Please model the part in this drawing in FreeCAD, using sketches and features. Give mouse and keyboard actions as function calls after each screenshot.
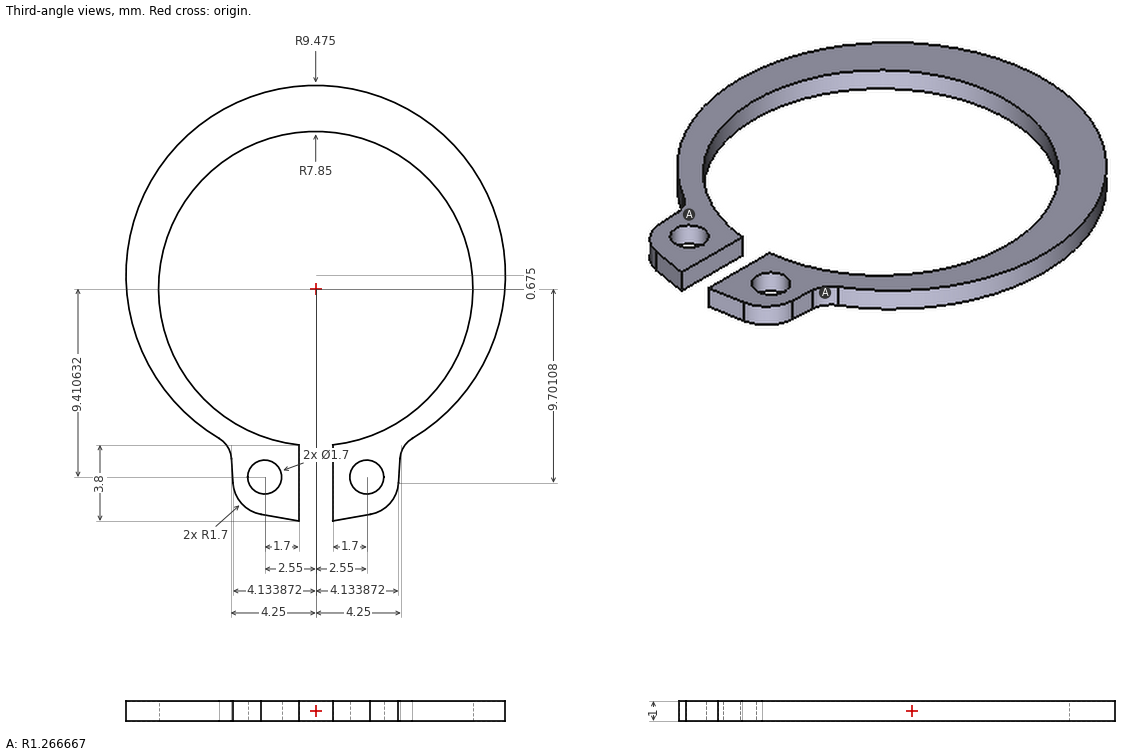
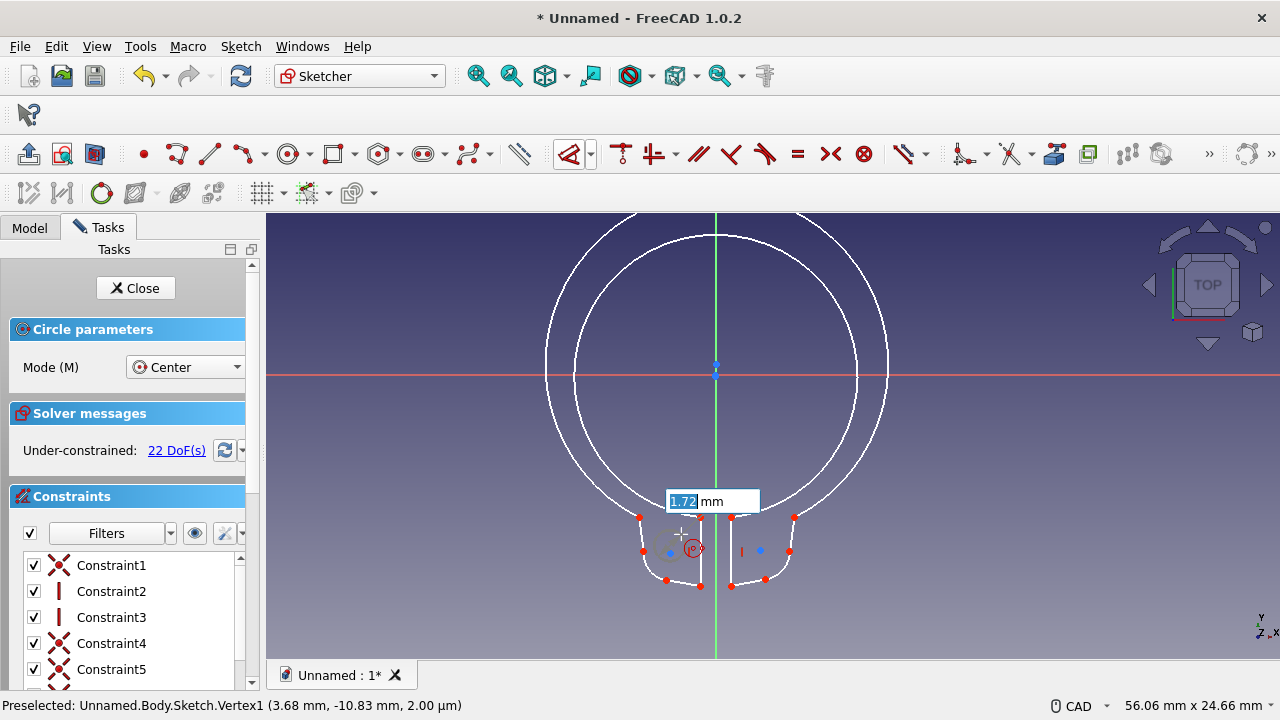
text(1.7)
key(Return)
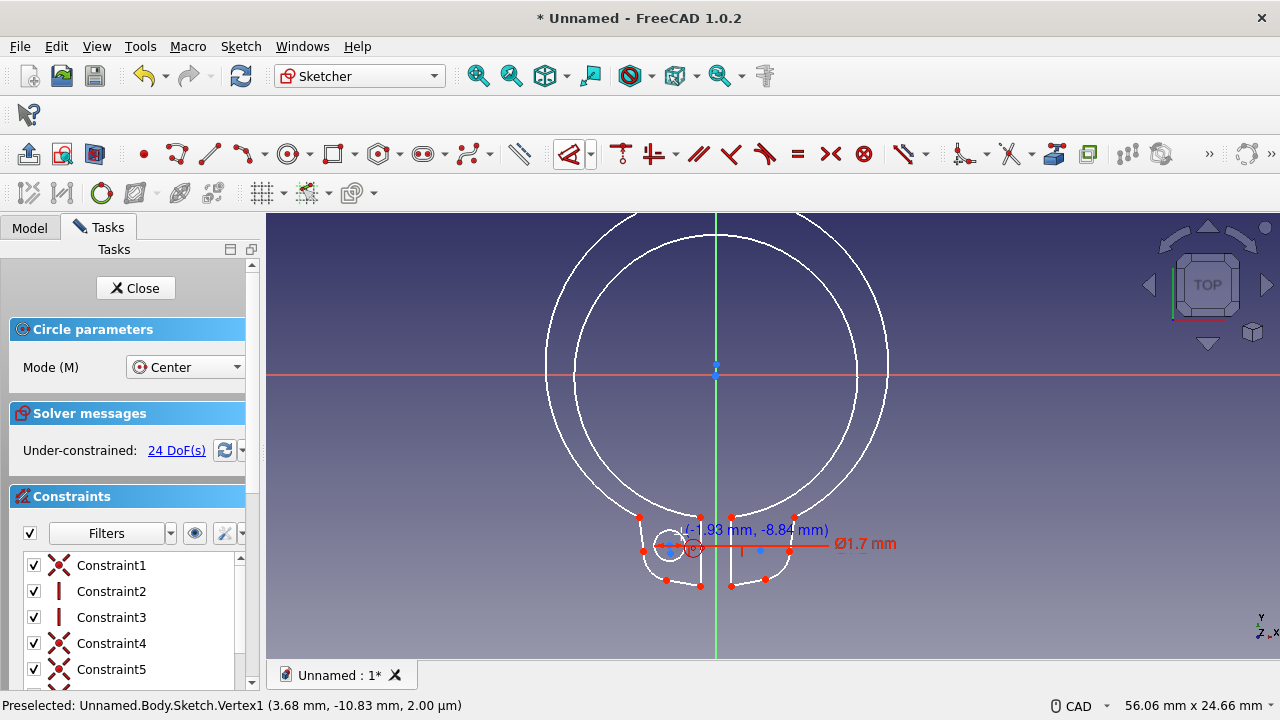
scroll(762, 545, up, 7)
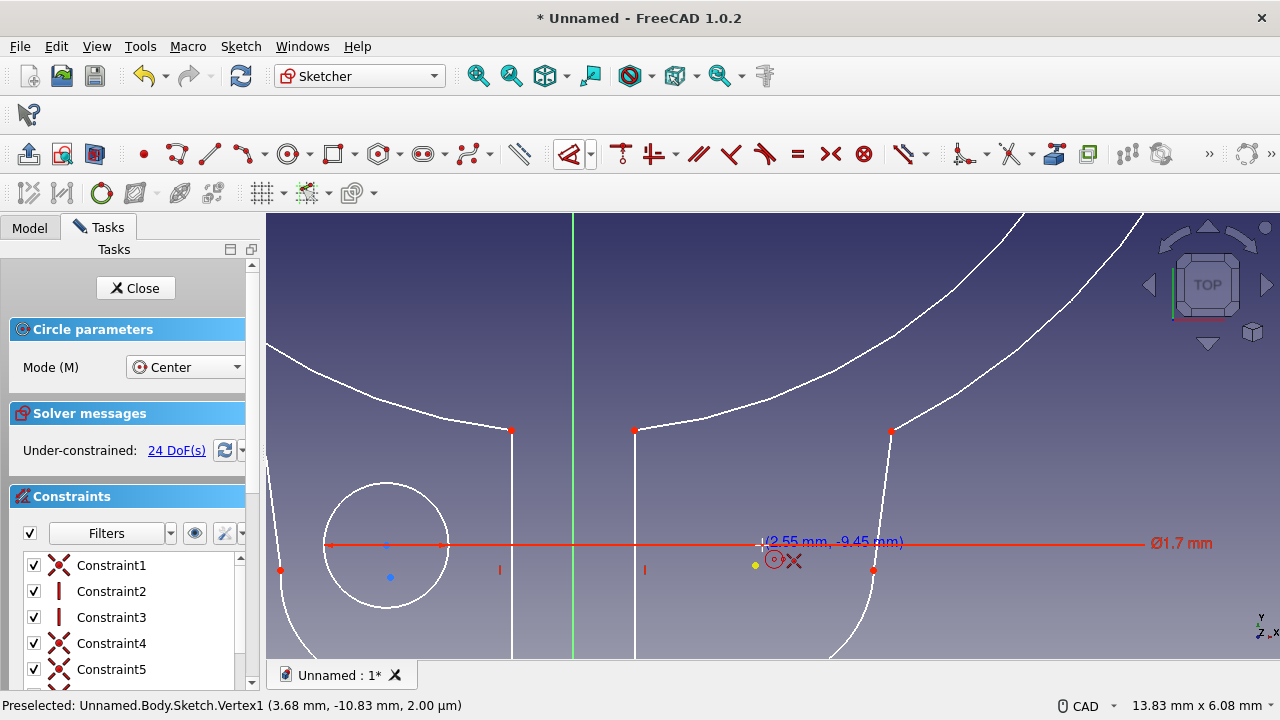
click(760, 544)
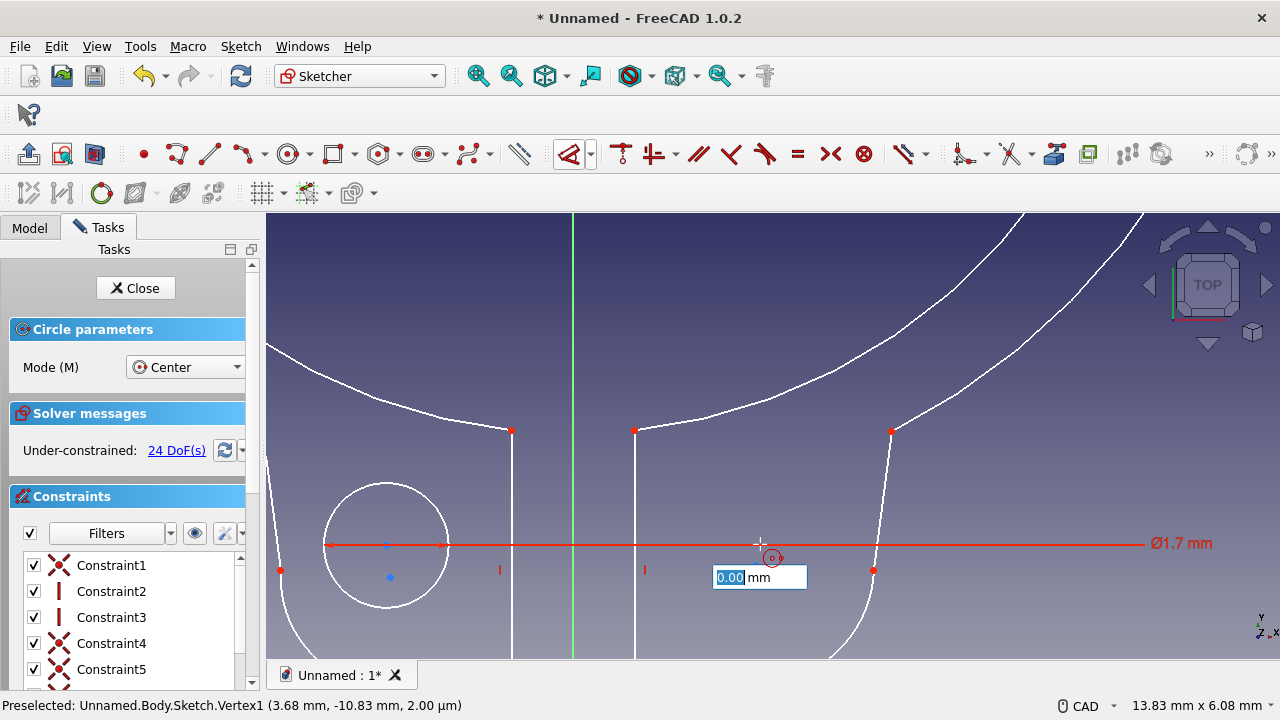
scroll(730, 541, down, 9)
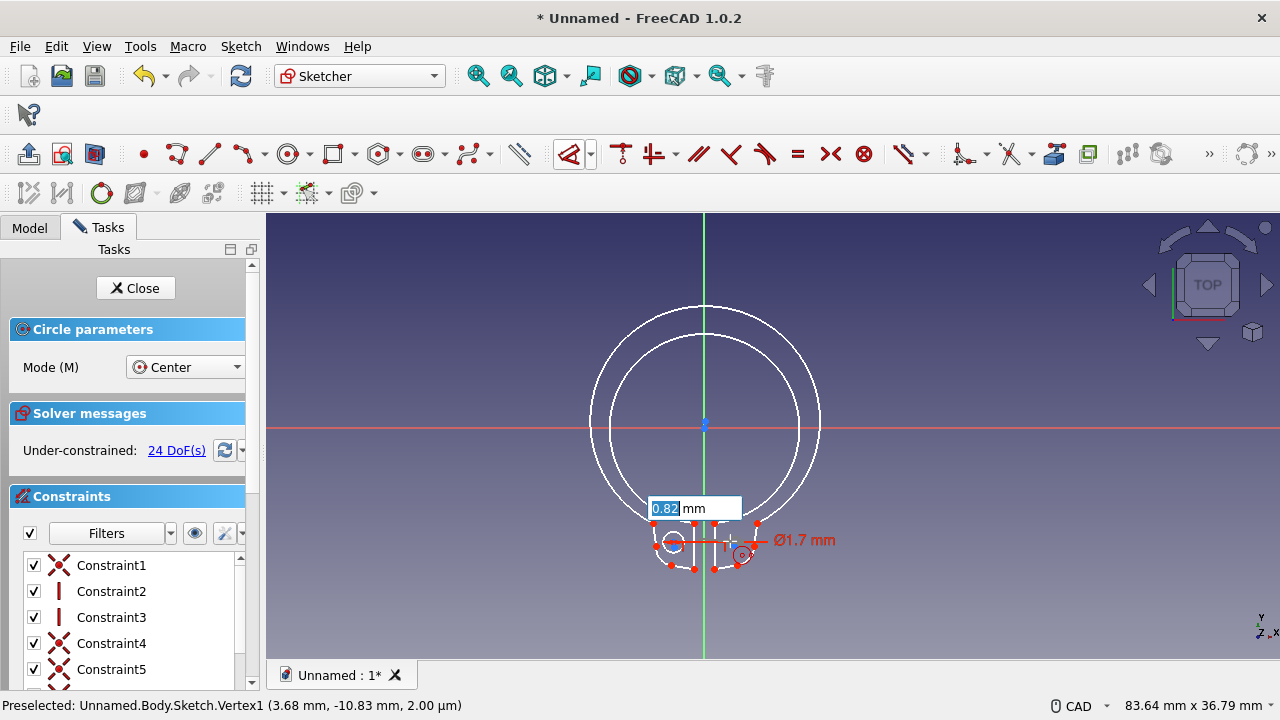
scroll(743, 535, up, 2)
move(742, 534)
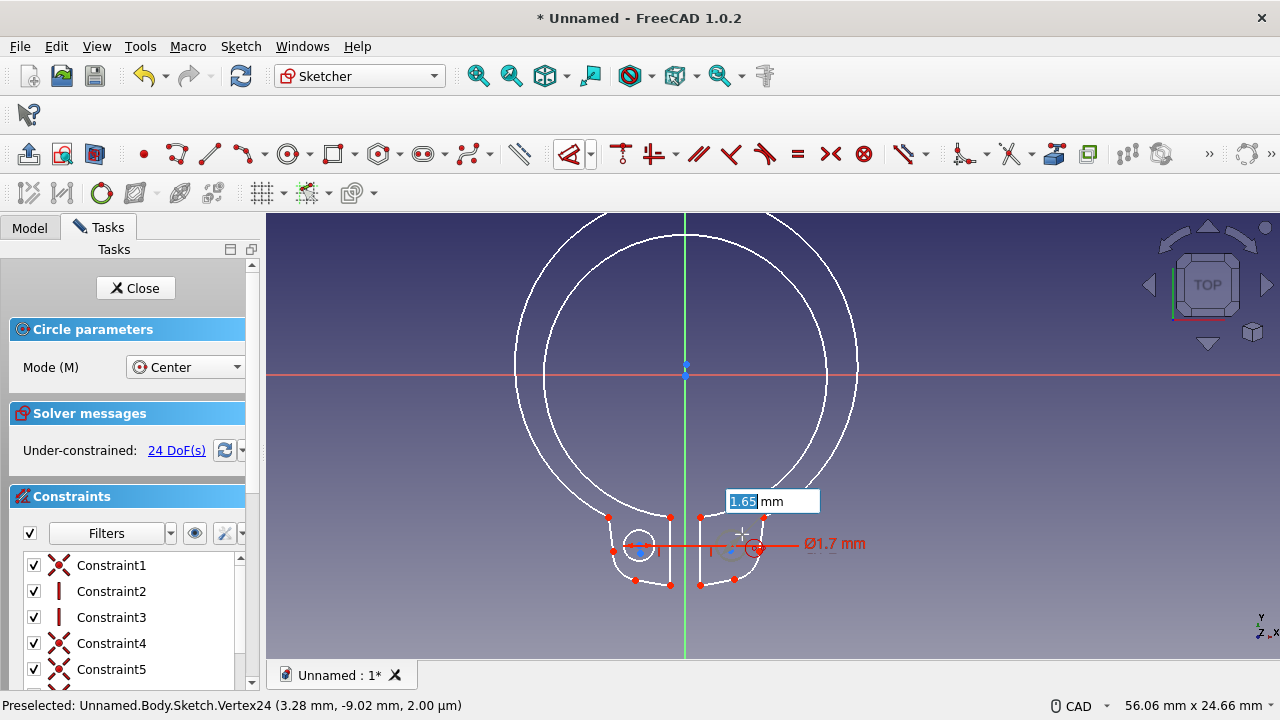
text(1.7)
key(Return)
key(Escape)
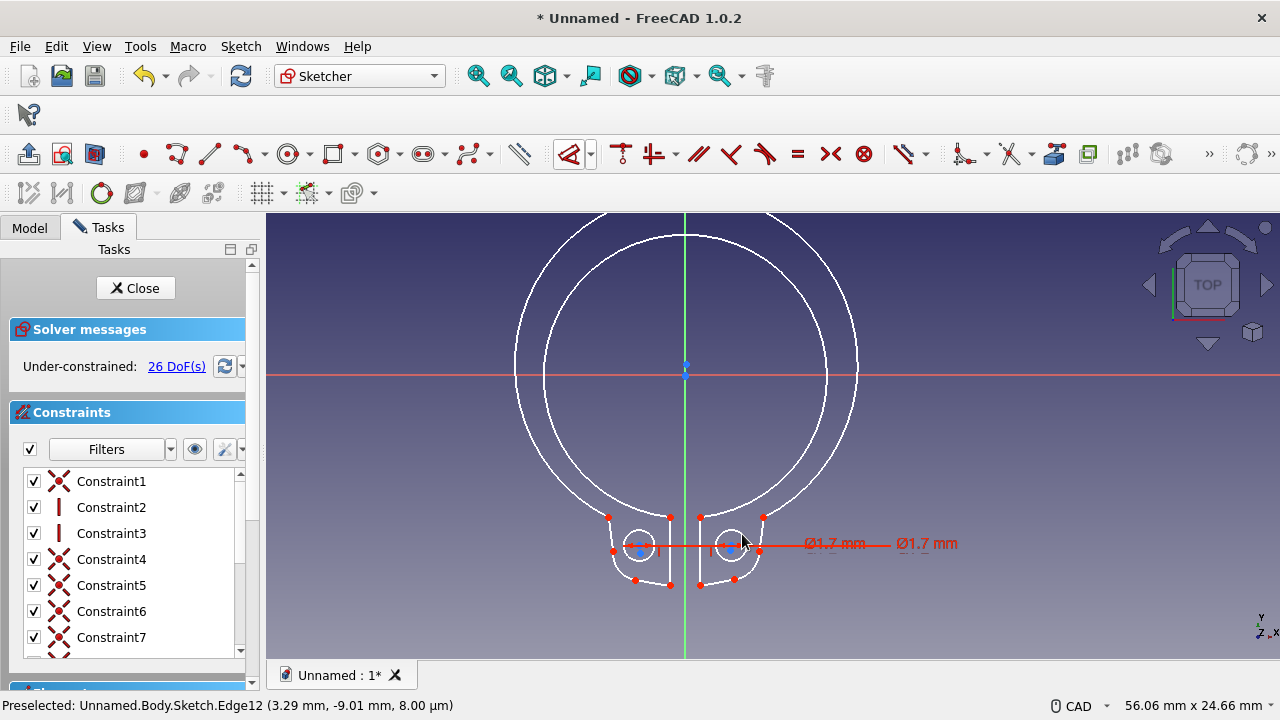
scroll(761, 542, up, 2)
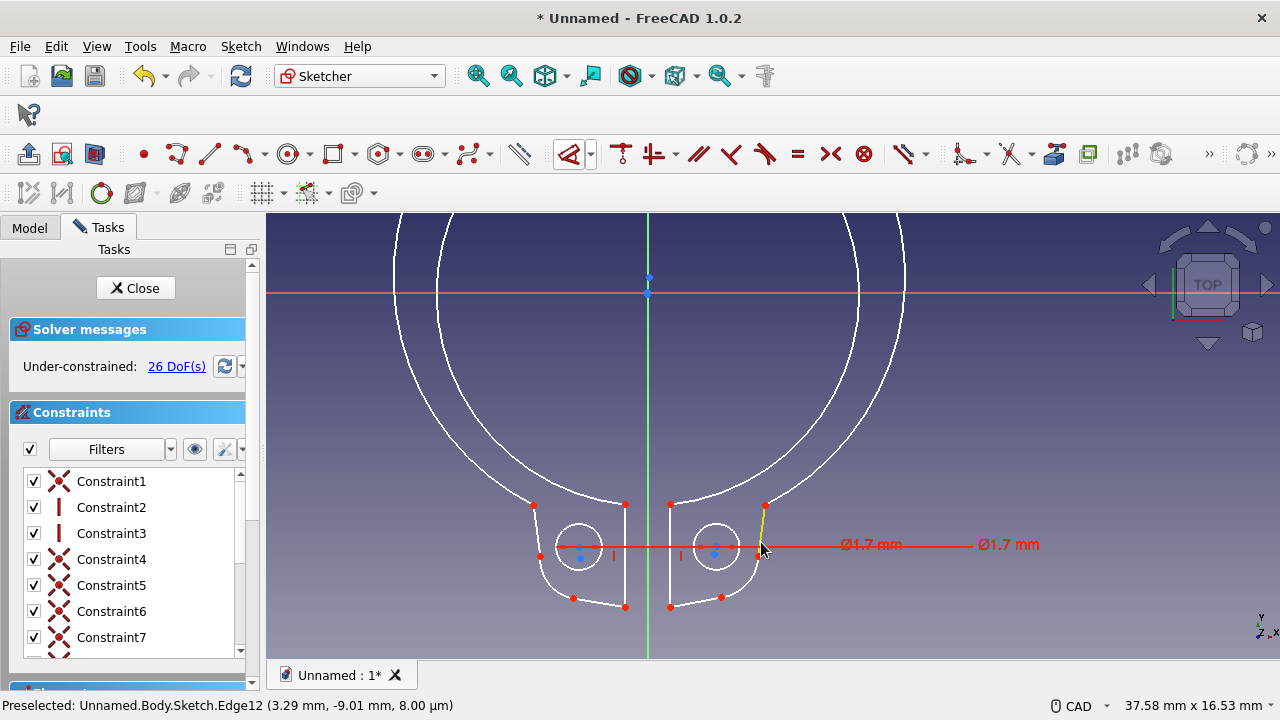
click(760, 541)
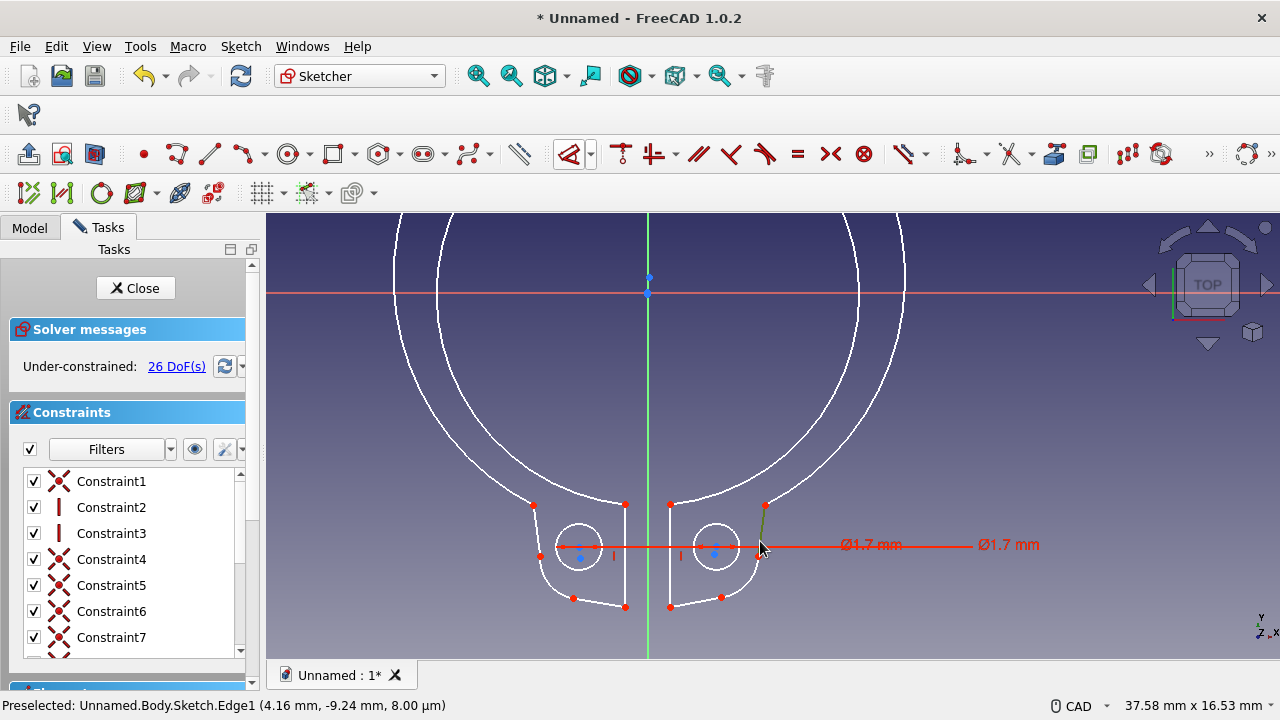
click(738, 591)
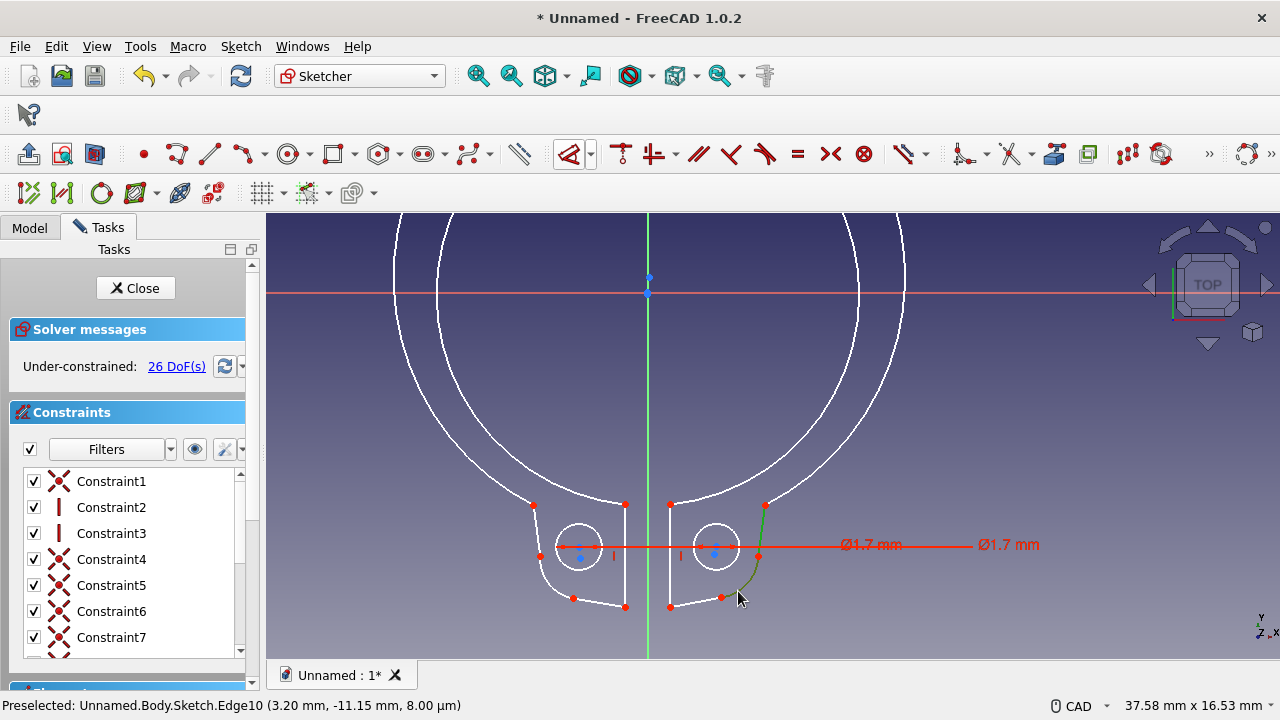
click(765, 154)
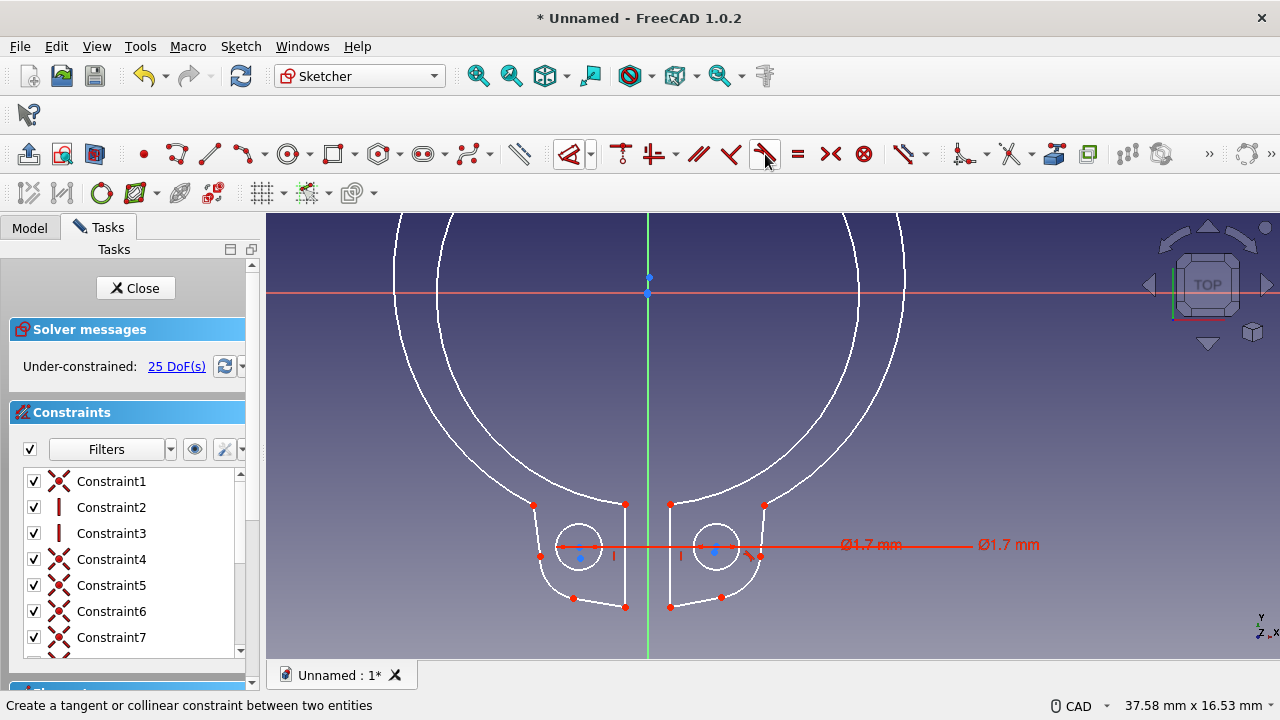
click(536, 520)